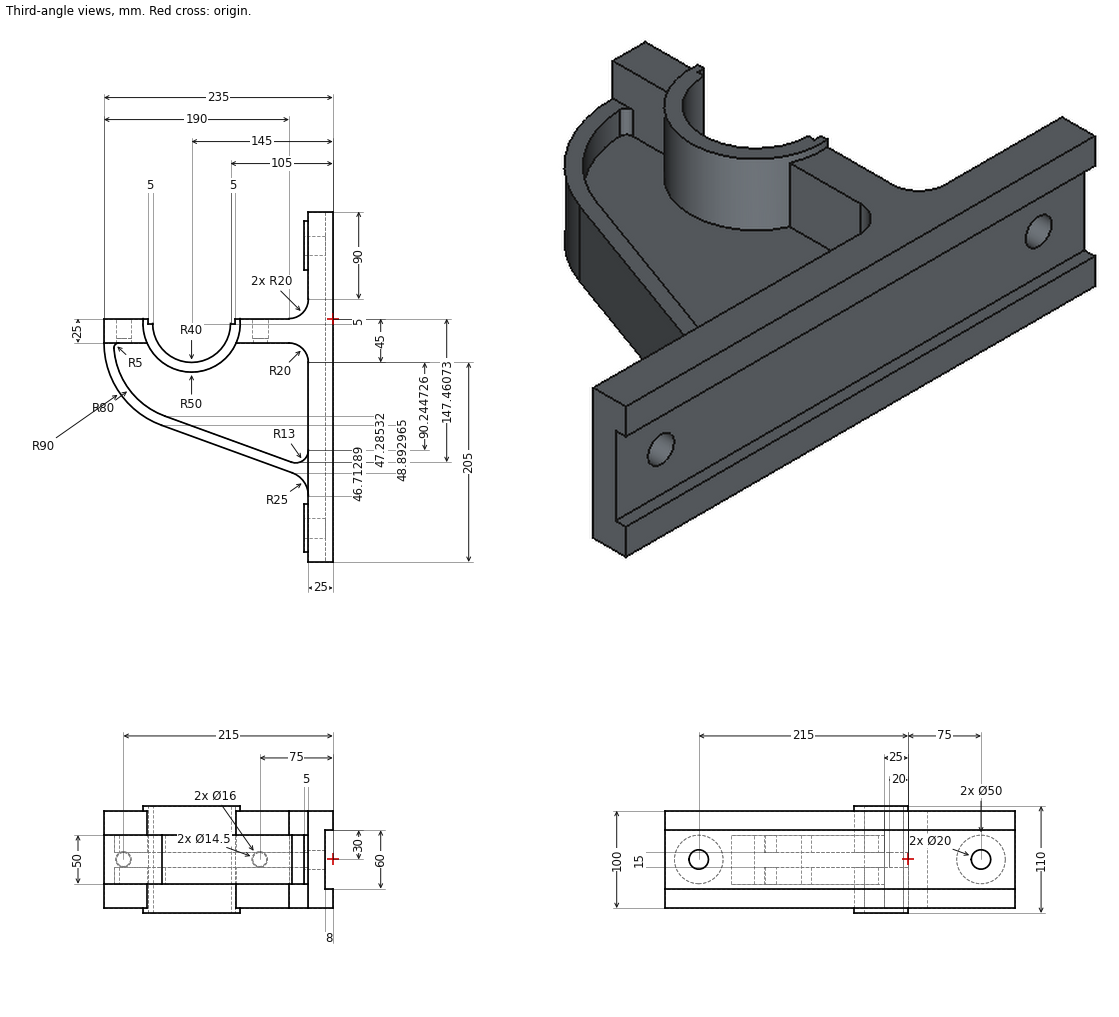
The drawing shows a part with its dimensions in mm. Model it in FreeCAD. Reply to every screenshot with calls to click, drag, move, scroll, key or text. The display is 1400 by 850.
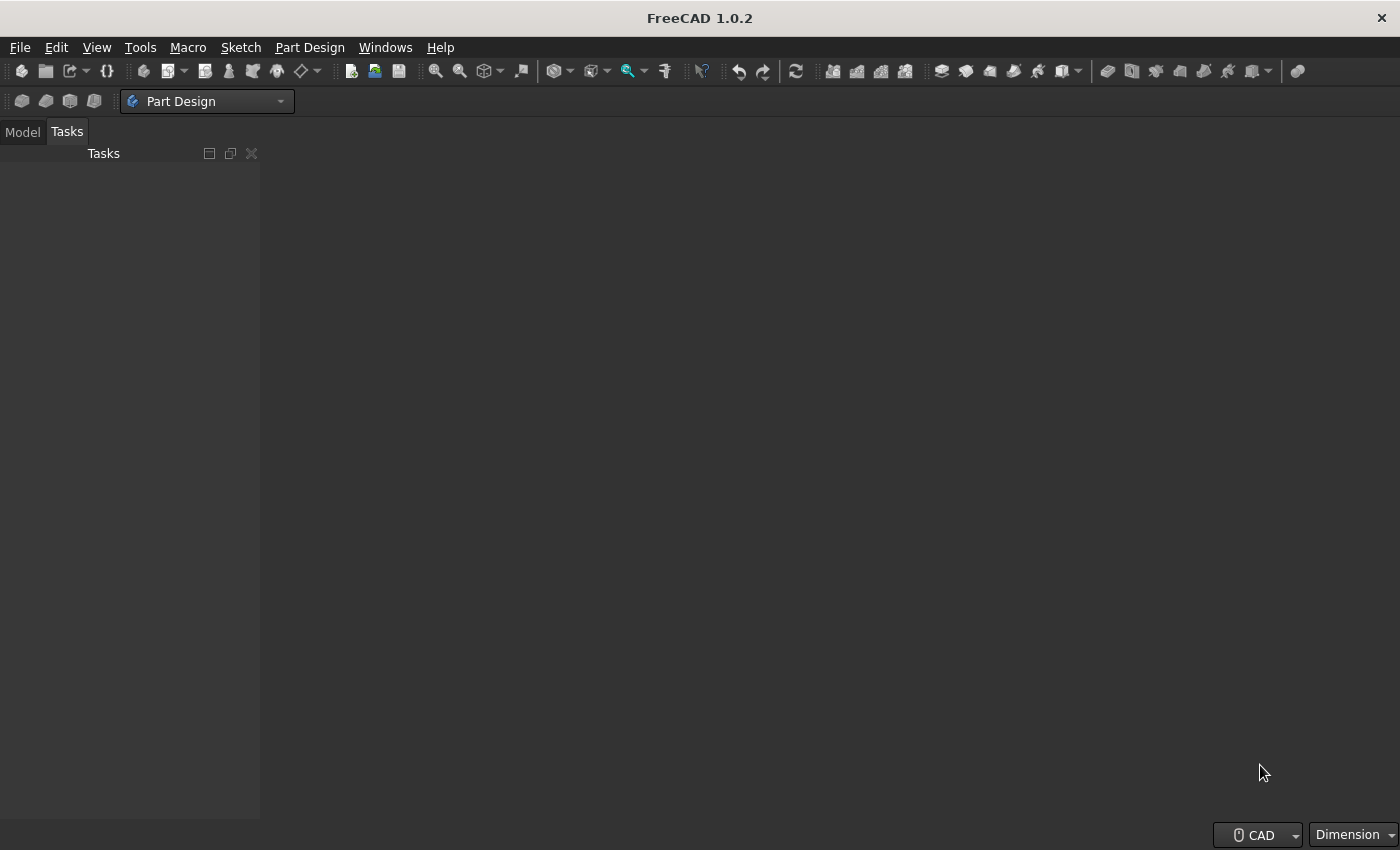
click(352, 72)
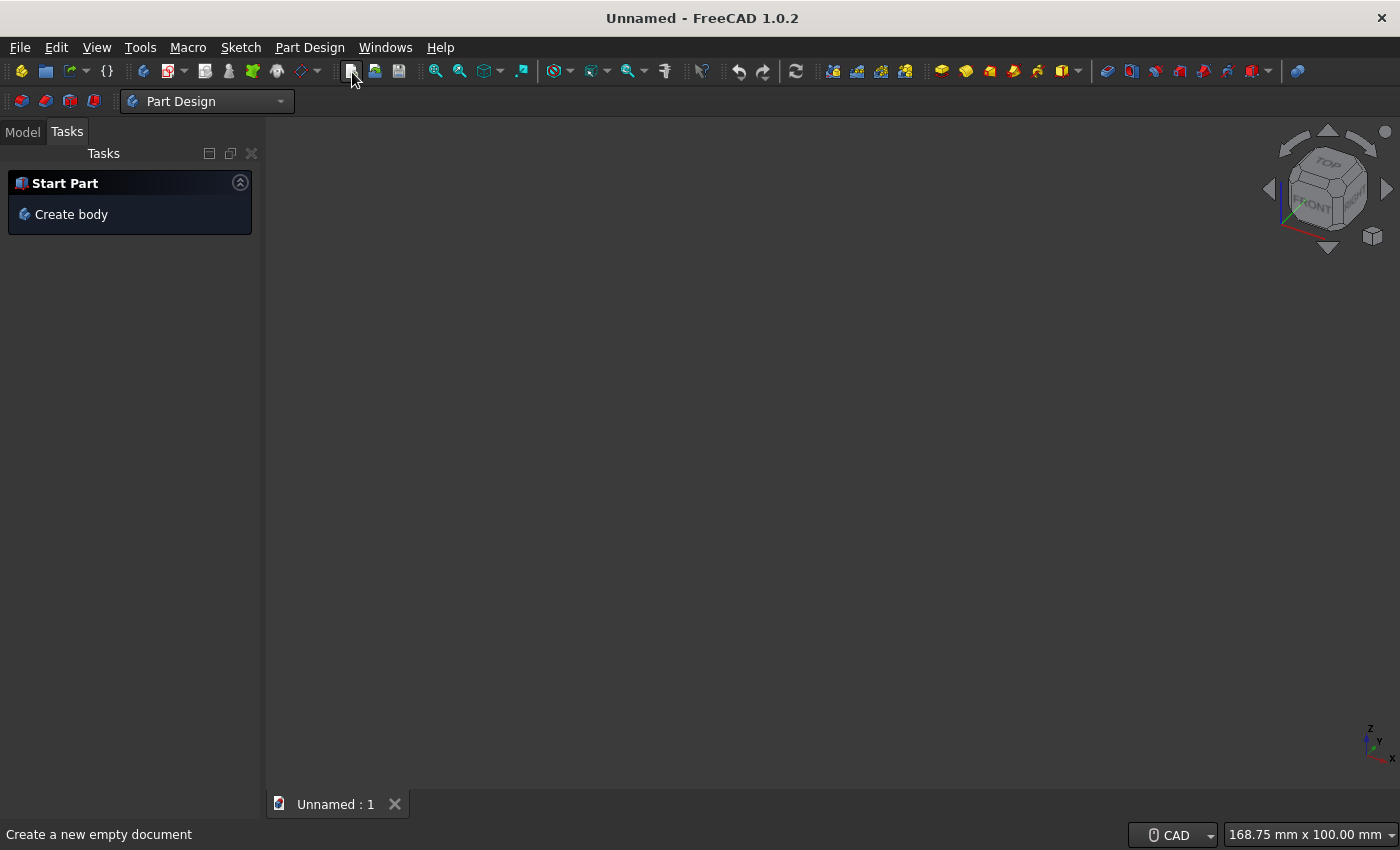
click(168, 72)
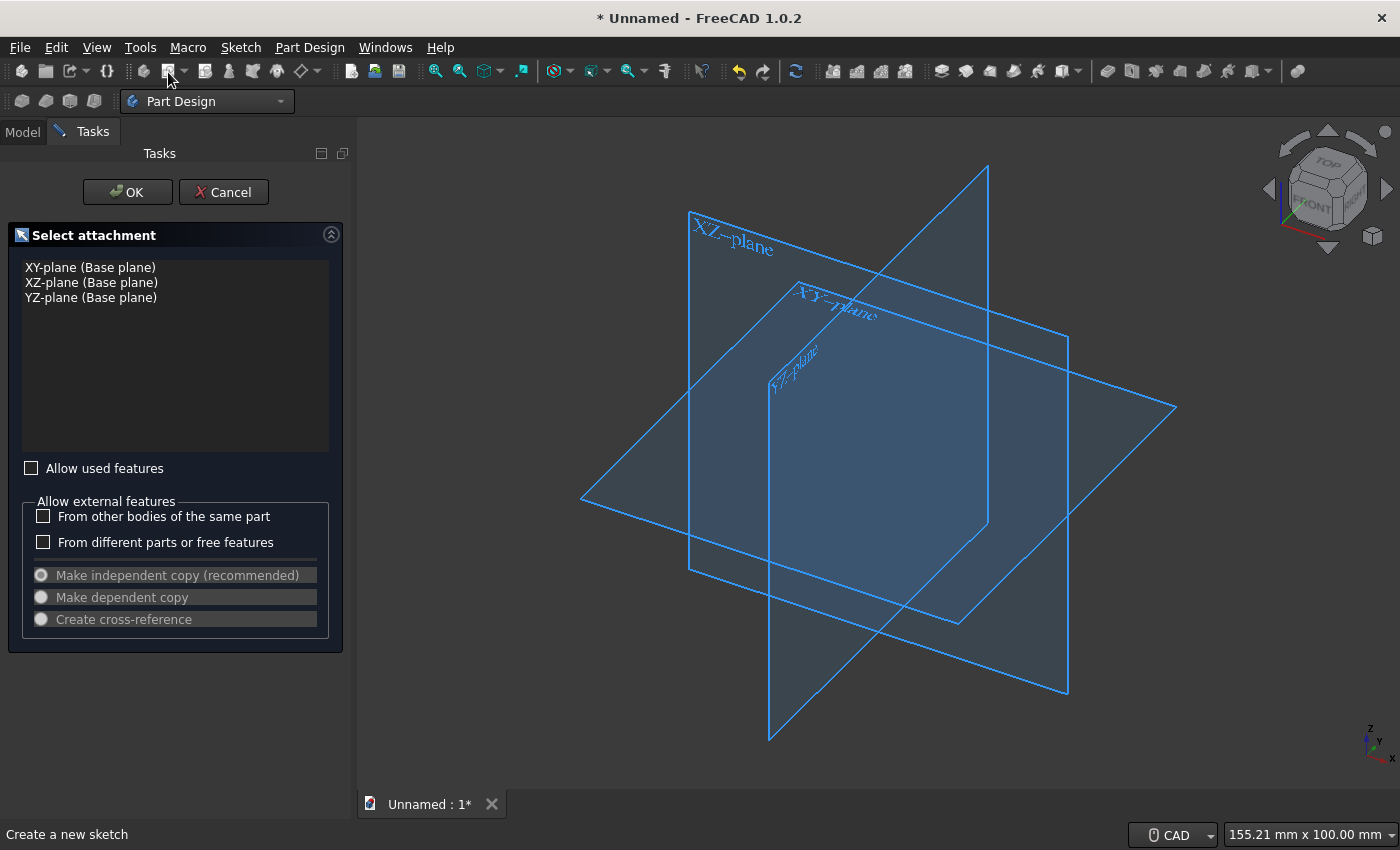
click(82, 268)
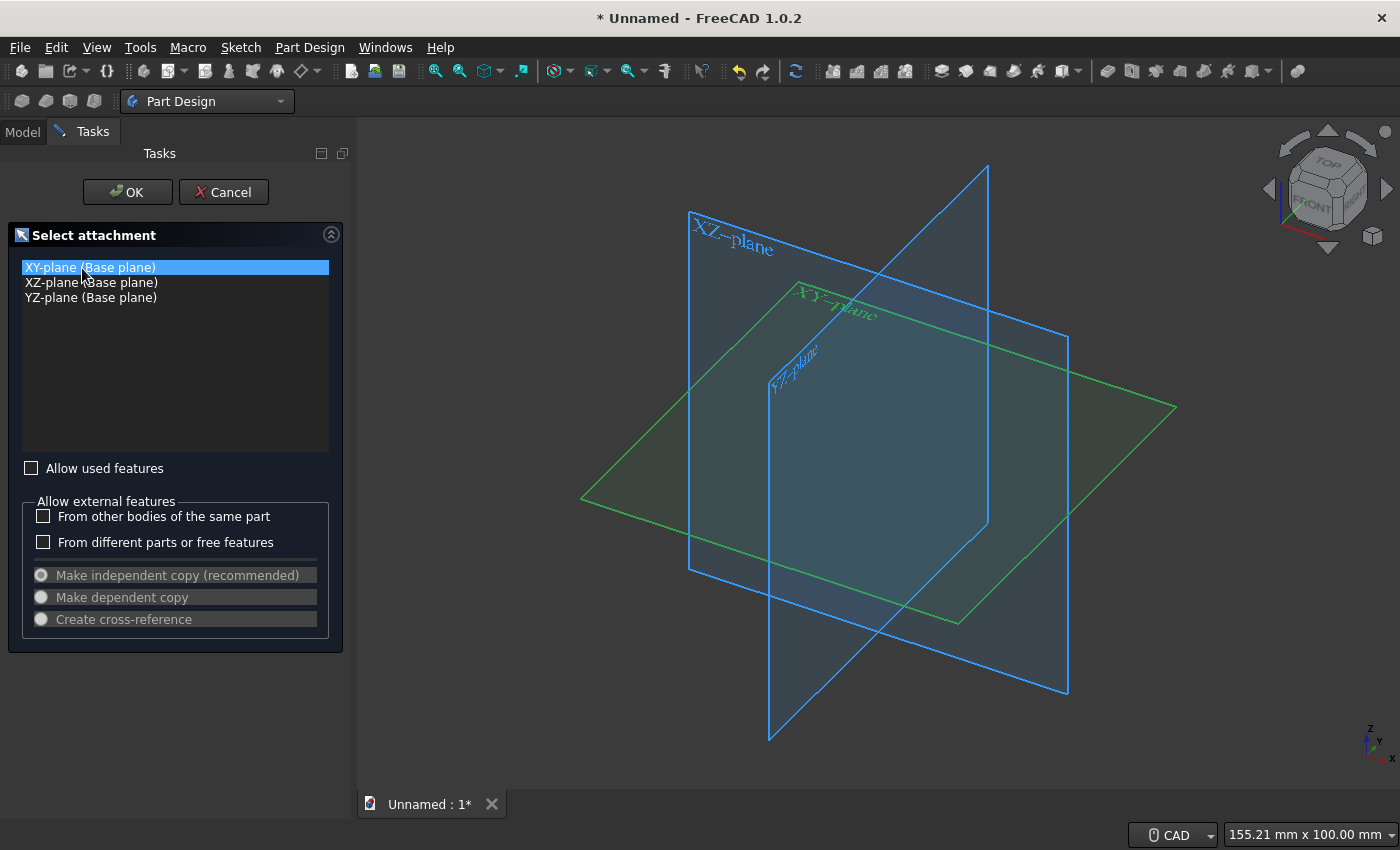
click(128, 192)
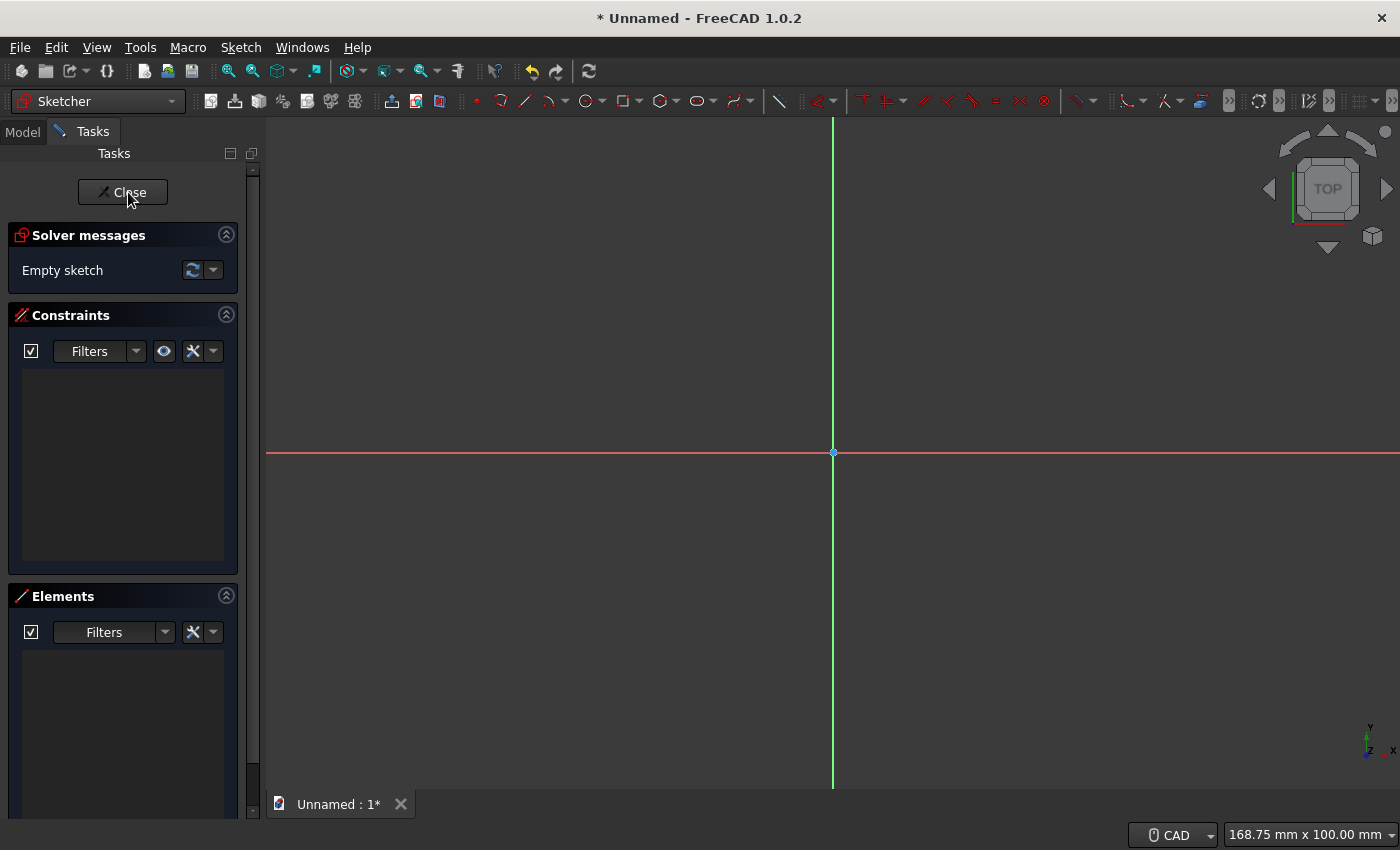
scroll(907, 360, down, 9)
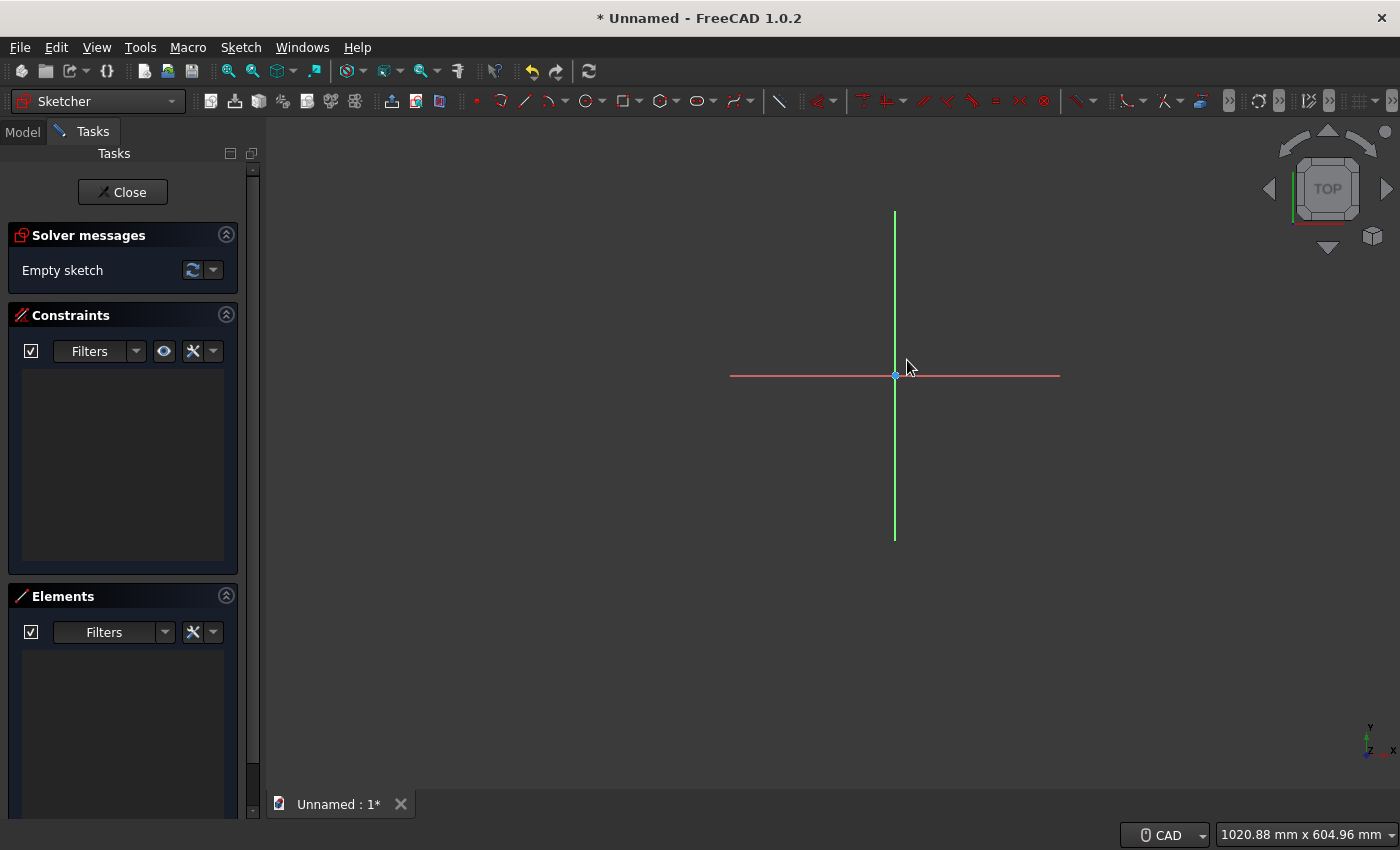
click(502, 102)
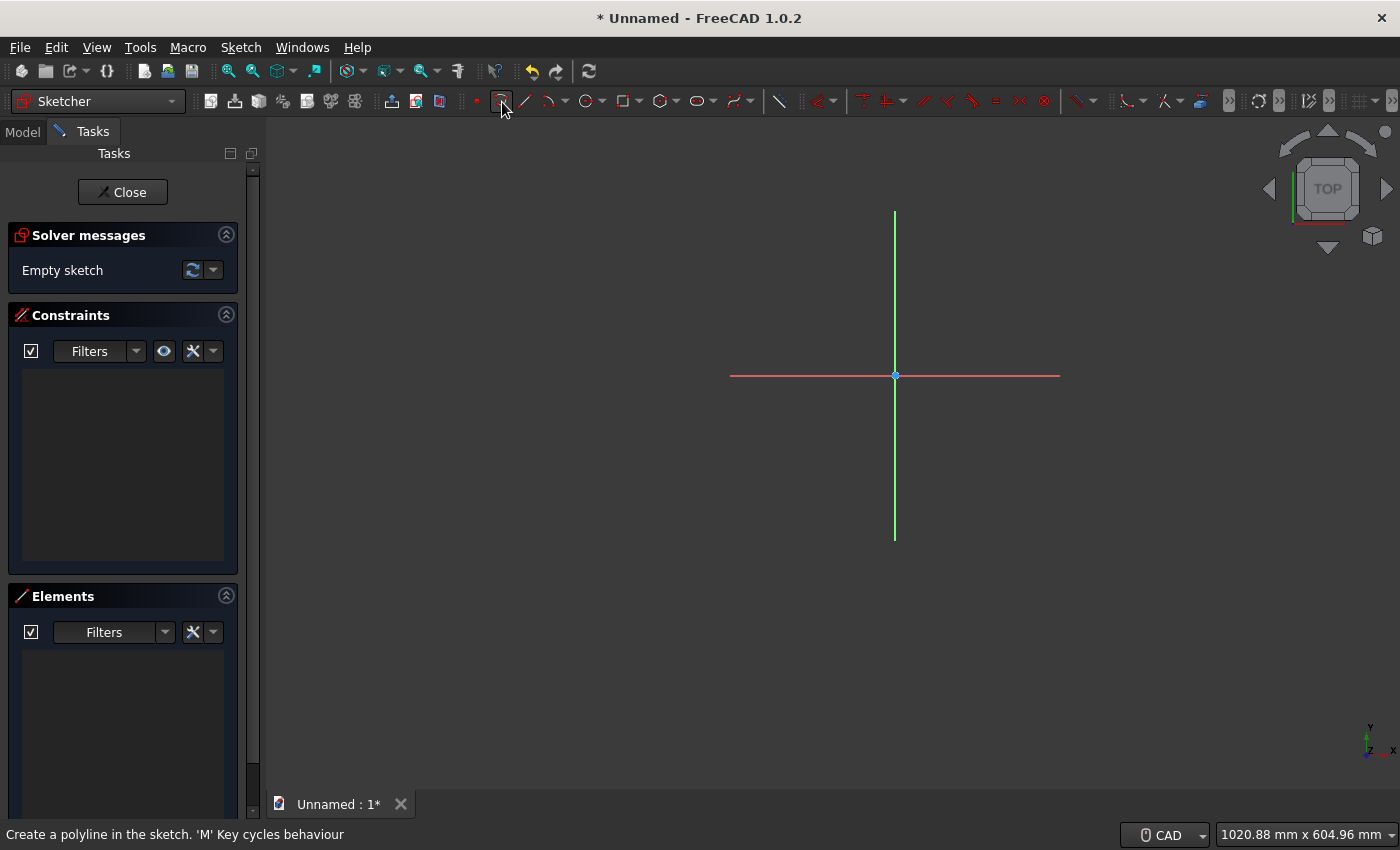
click(845, 376)
click(634, 385)
click(634, 403)
click(845, 403)
right_click(845, 403)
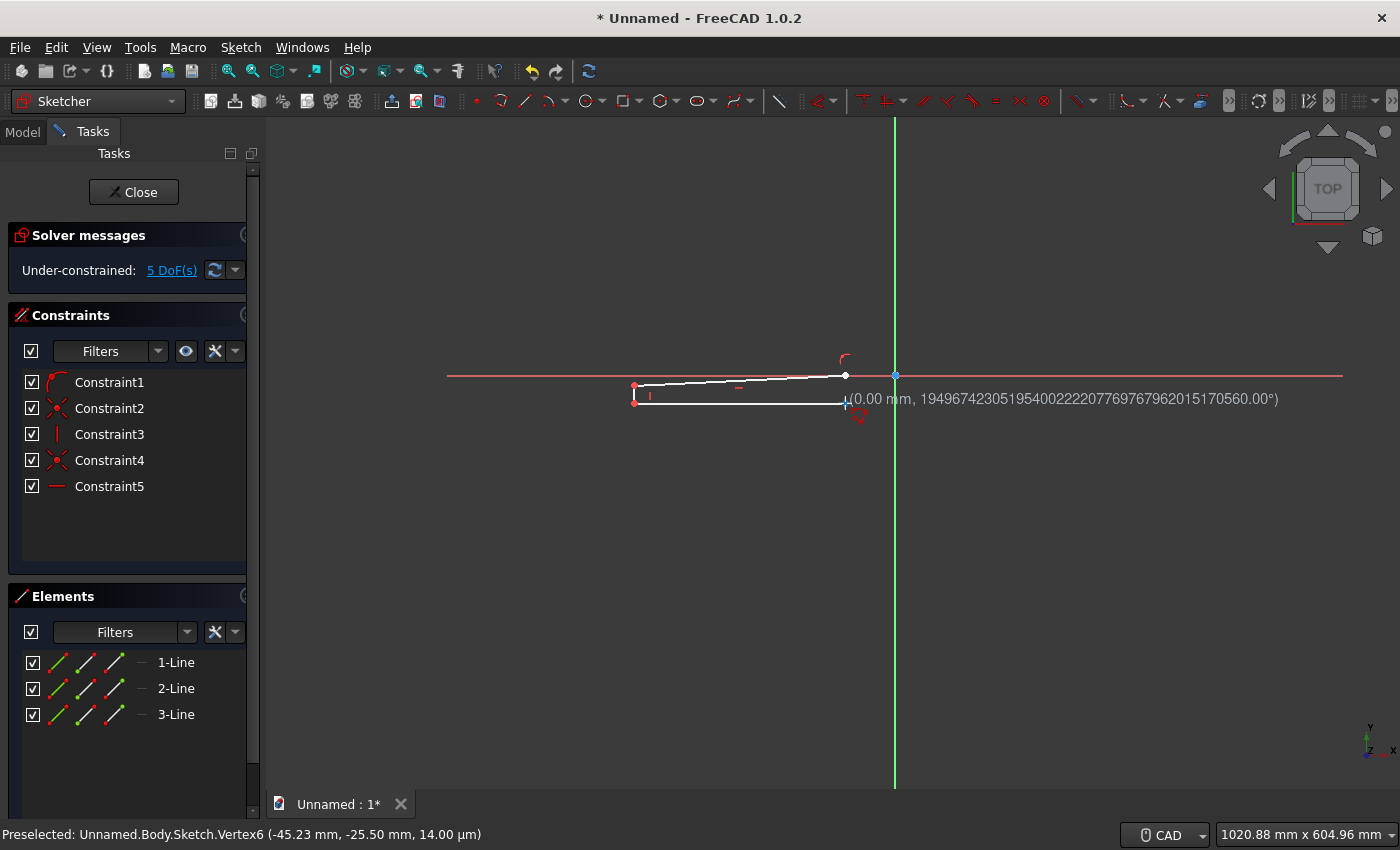
click(867, 426)
click(867, 653)
click(895, 653)
click(886, 253)
click(867, 253)
click(867, 353)
right_click(867, 353)